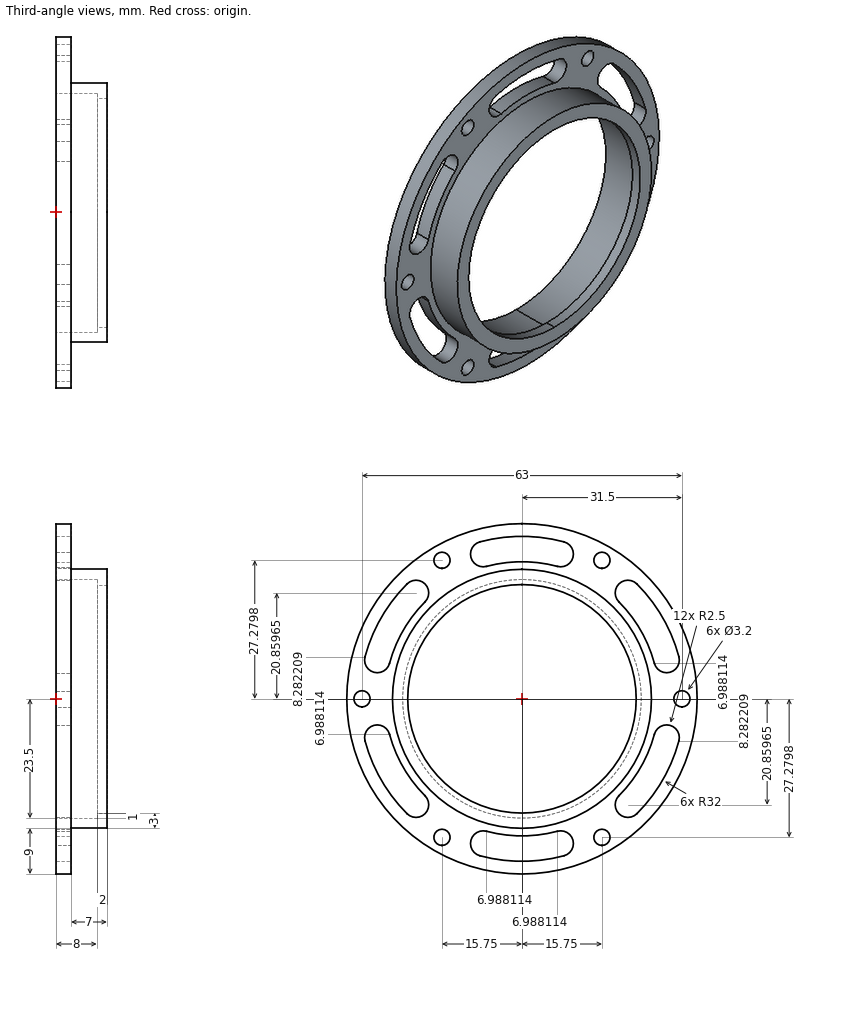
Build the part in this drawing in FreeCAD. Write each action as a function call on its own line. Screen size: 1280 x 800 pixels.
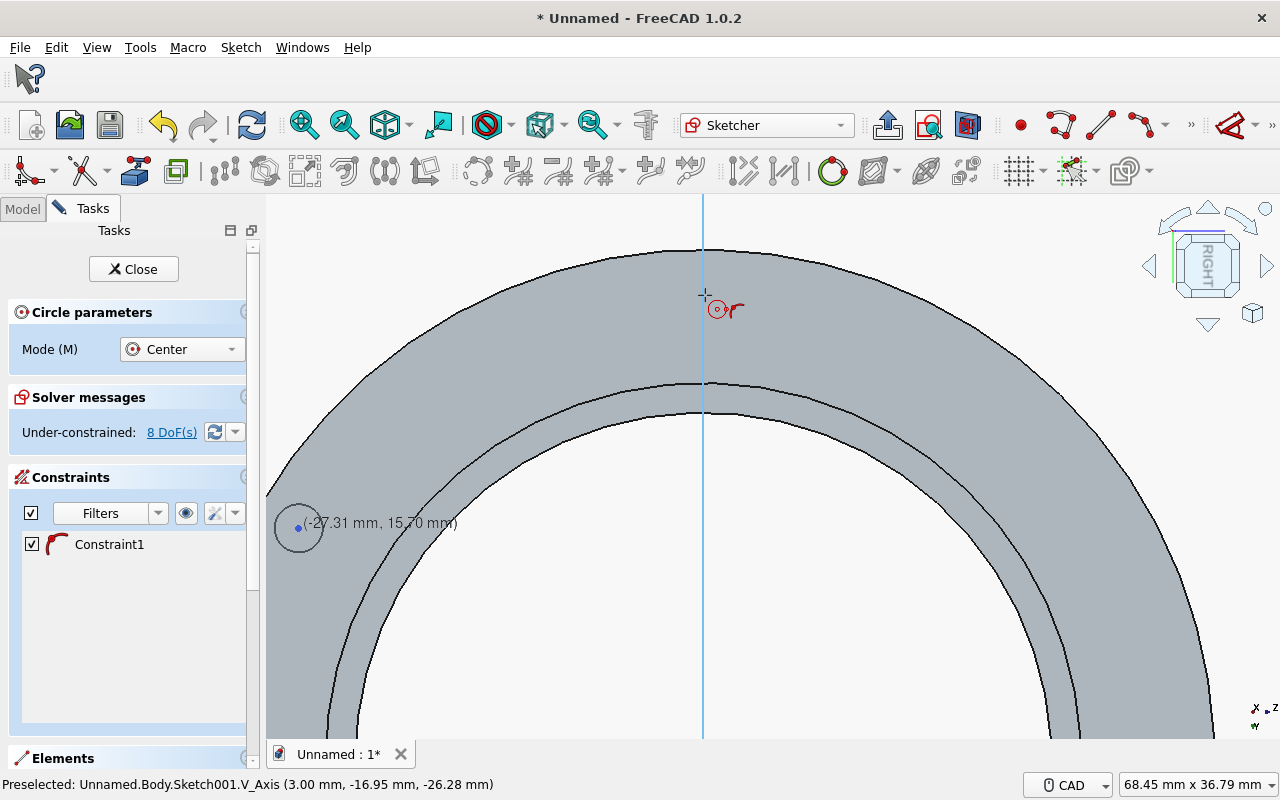
click(703, 294)
click(720, 277)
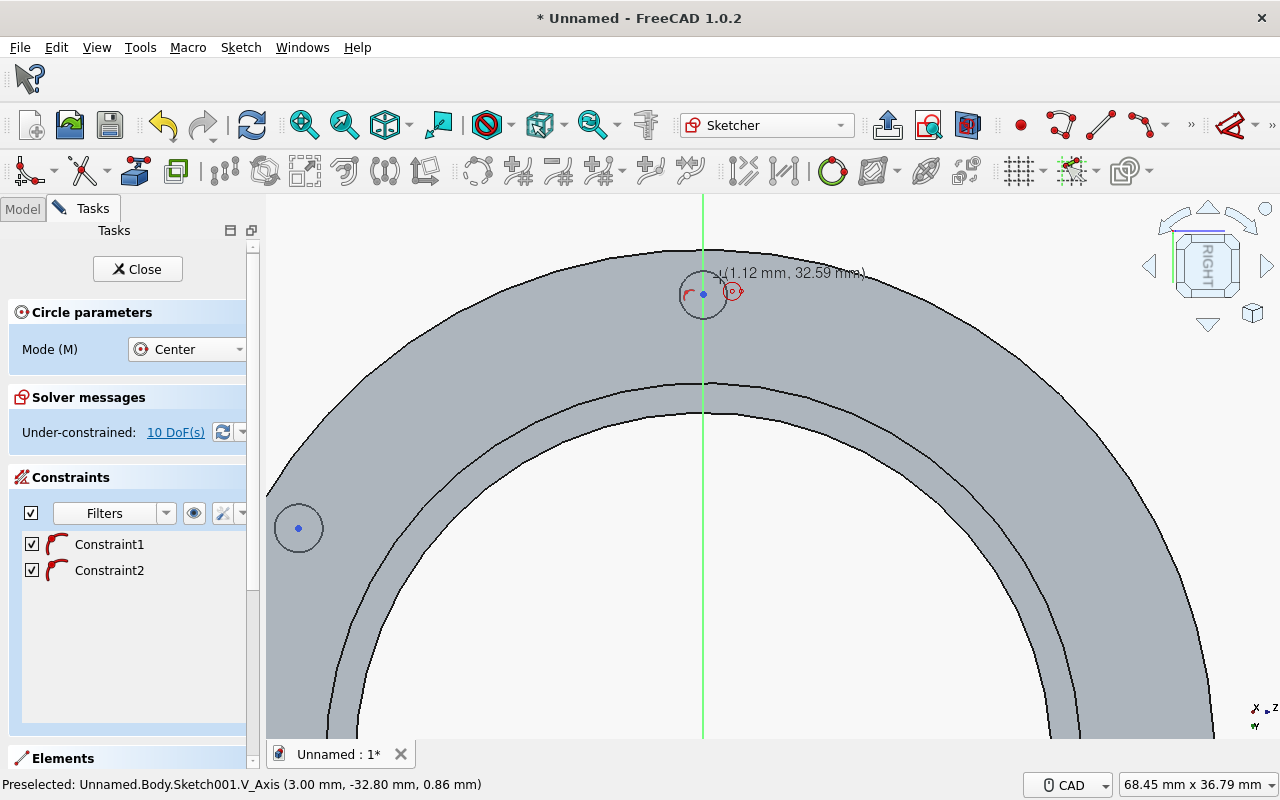
click(1107, 528)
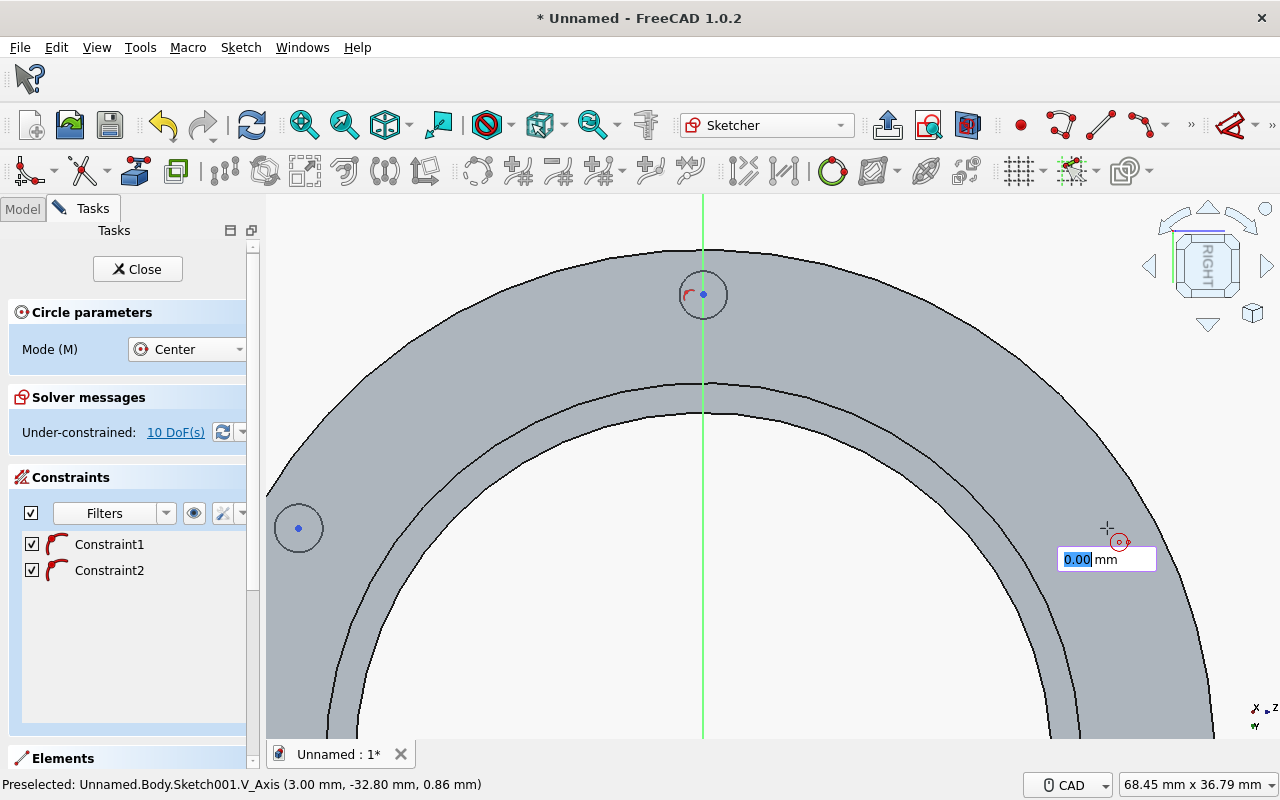
scroll(705, 295, down, 5)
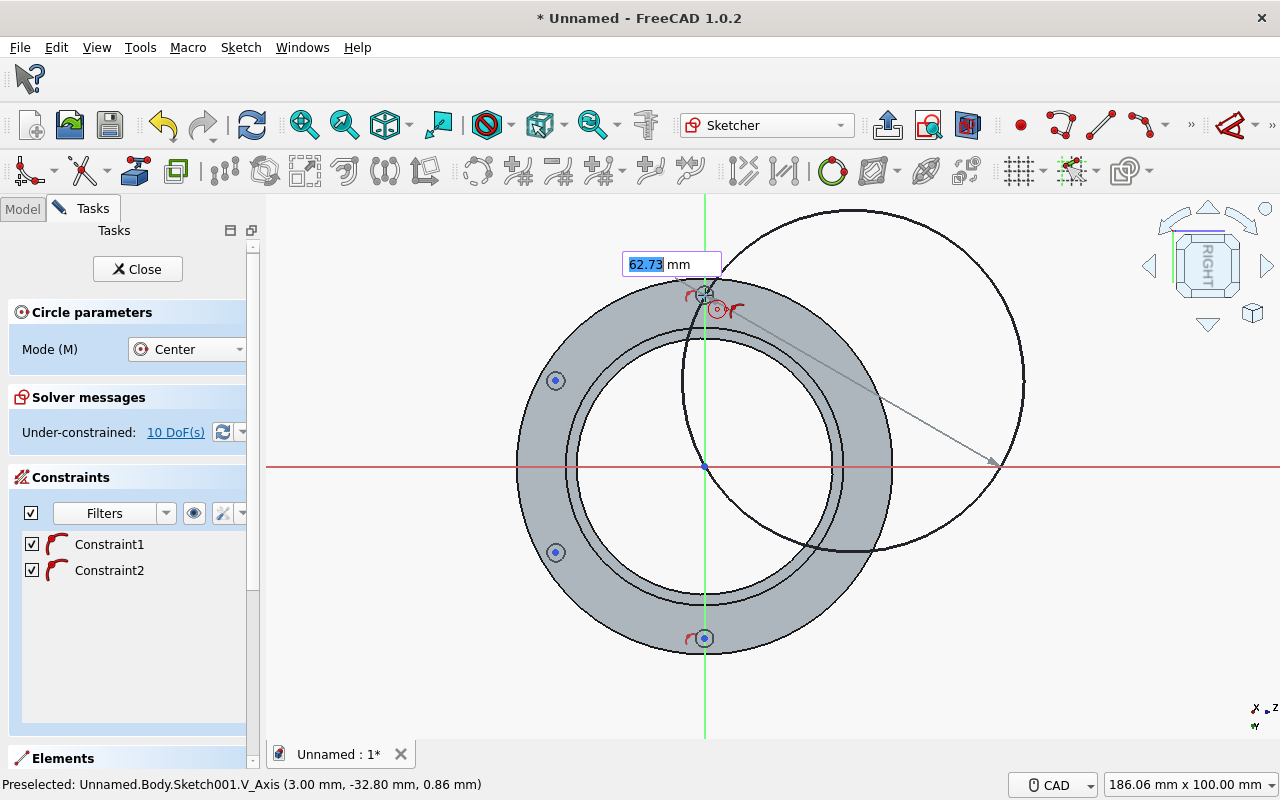
scroll(860, 374, up, 3)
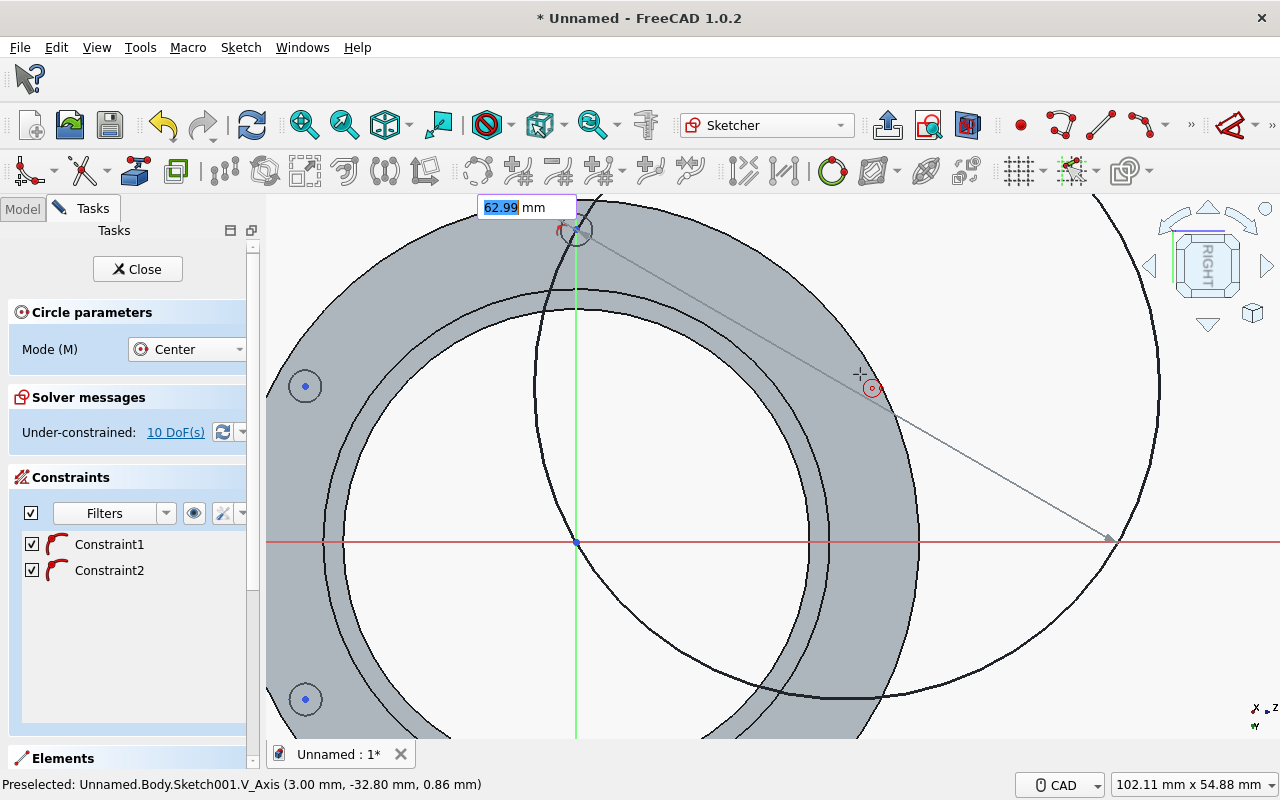
click(859, 375)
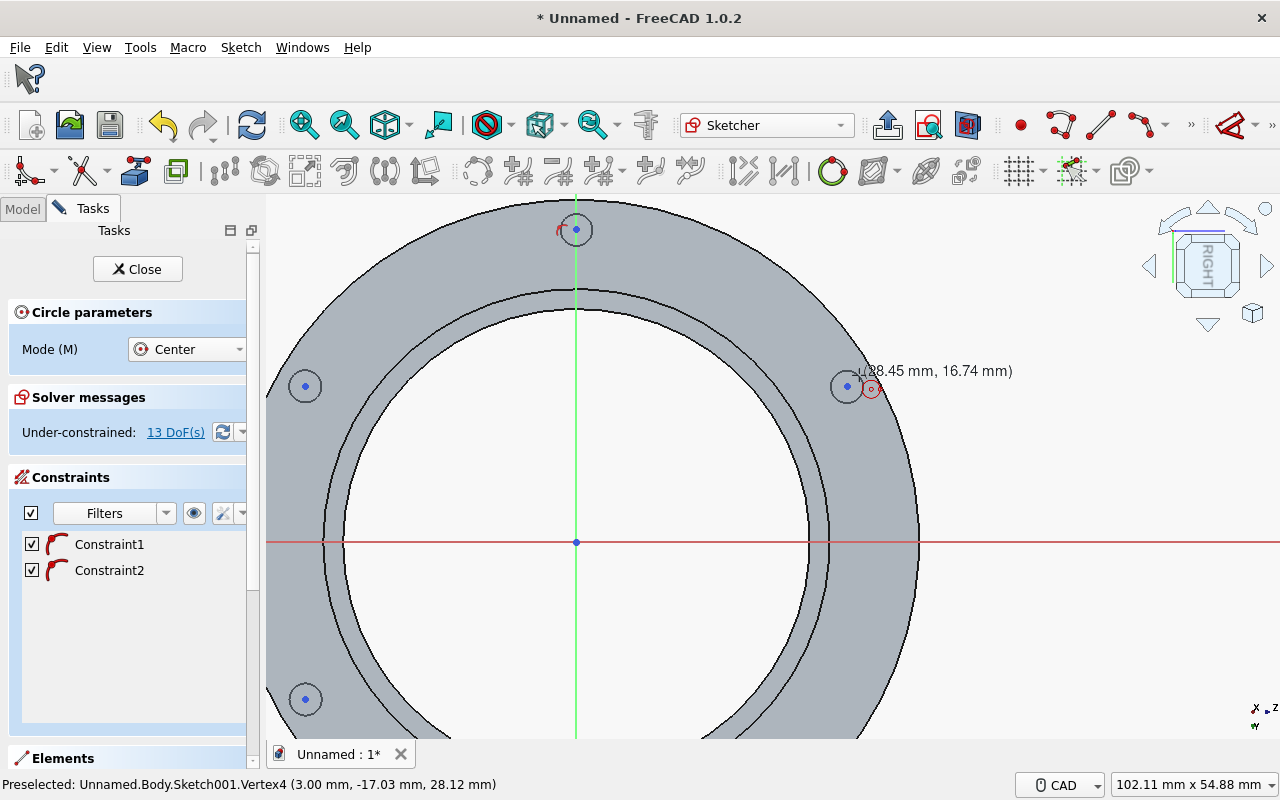
scroll(847, 699, up, 2)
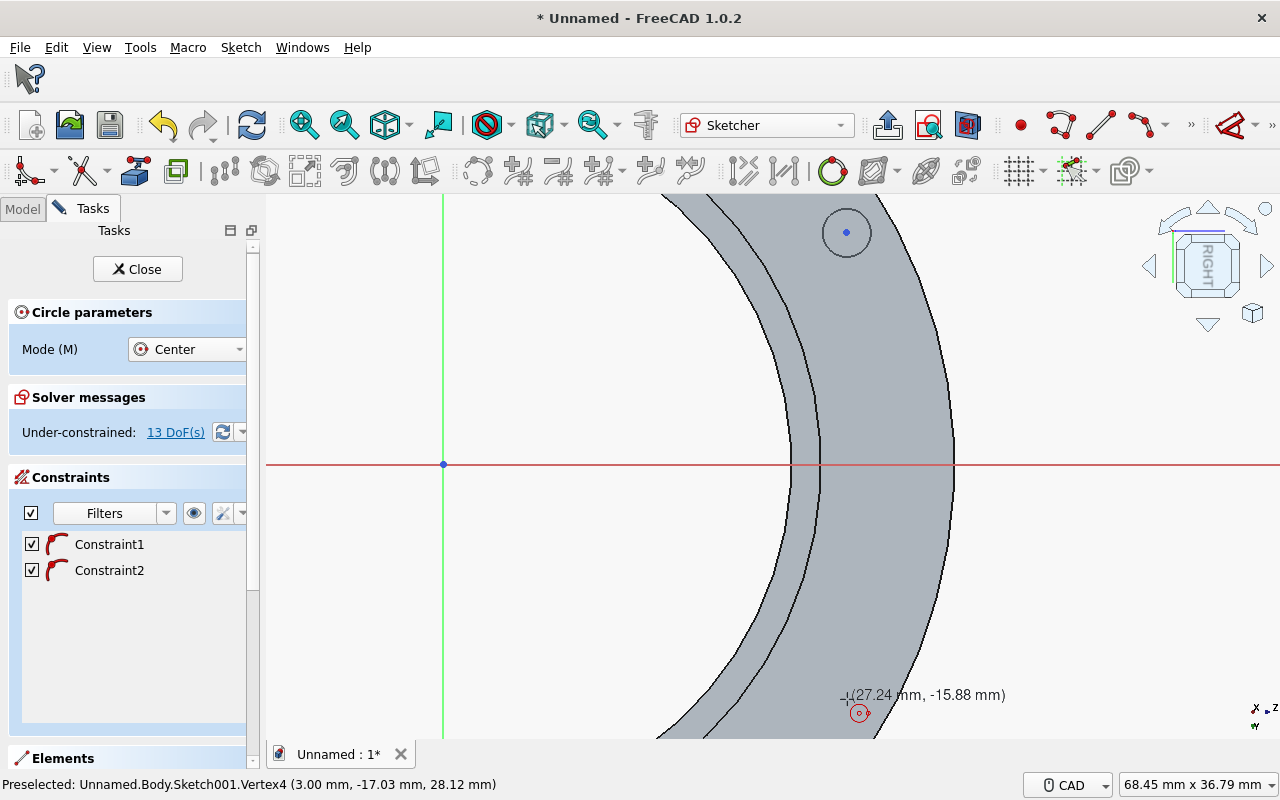
click(847, 698)
click(864, 681)
key(Escape)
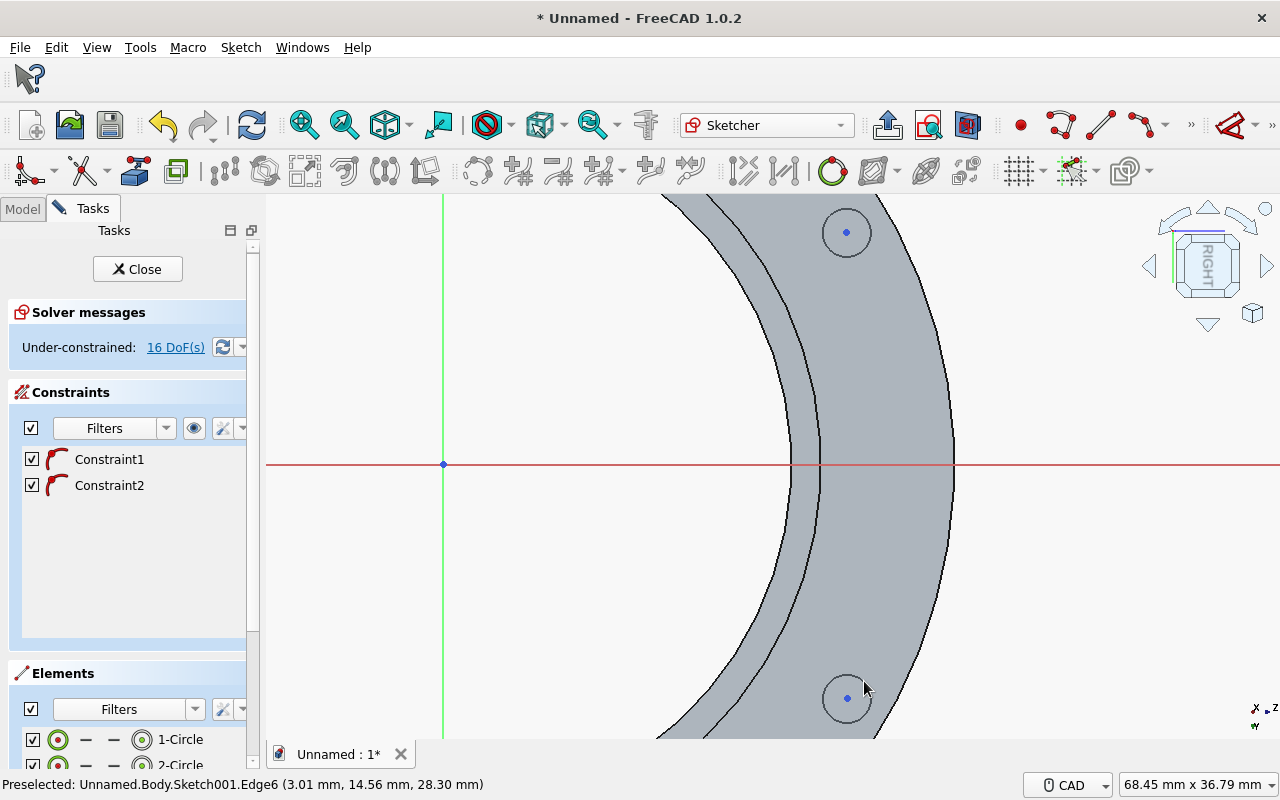
scroll(857, 468, down, 5)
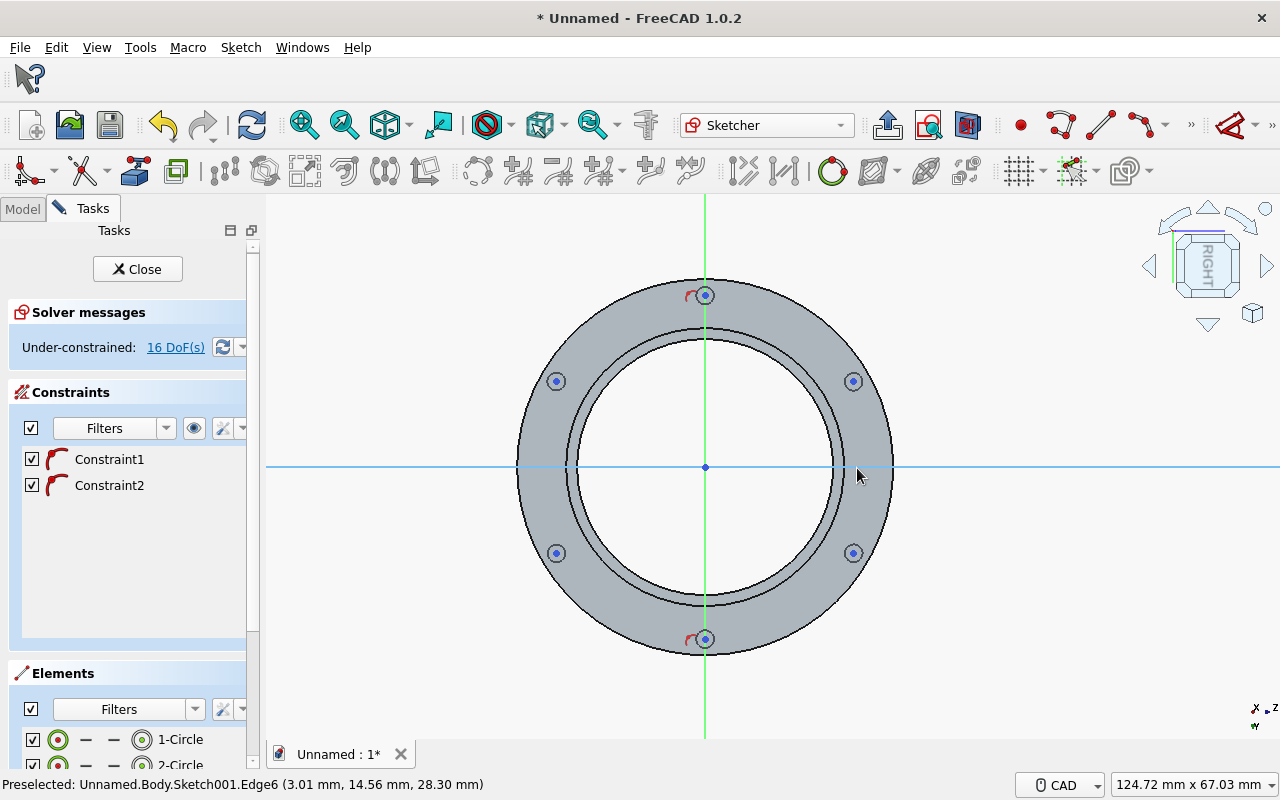
scroll(711, 633, up, 4)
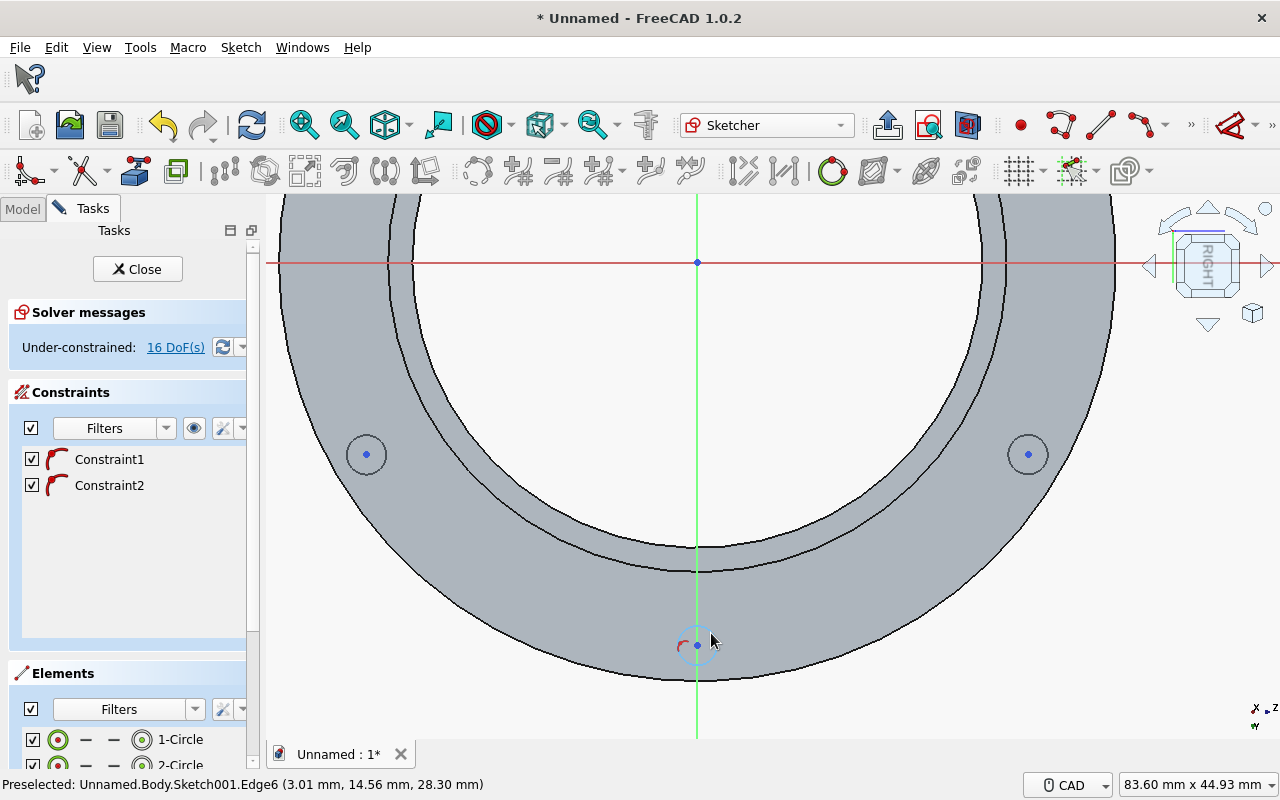
click(711, 632)